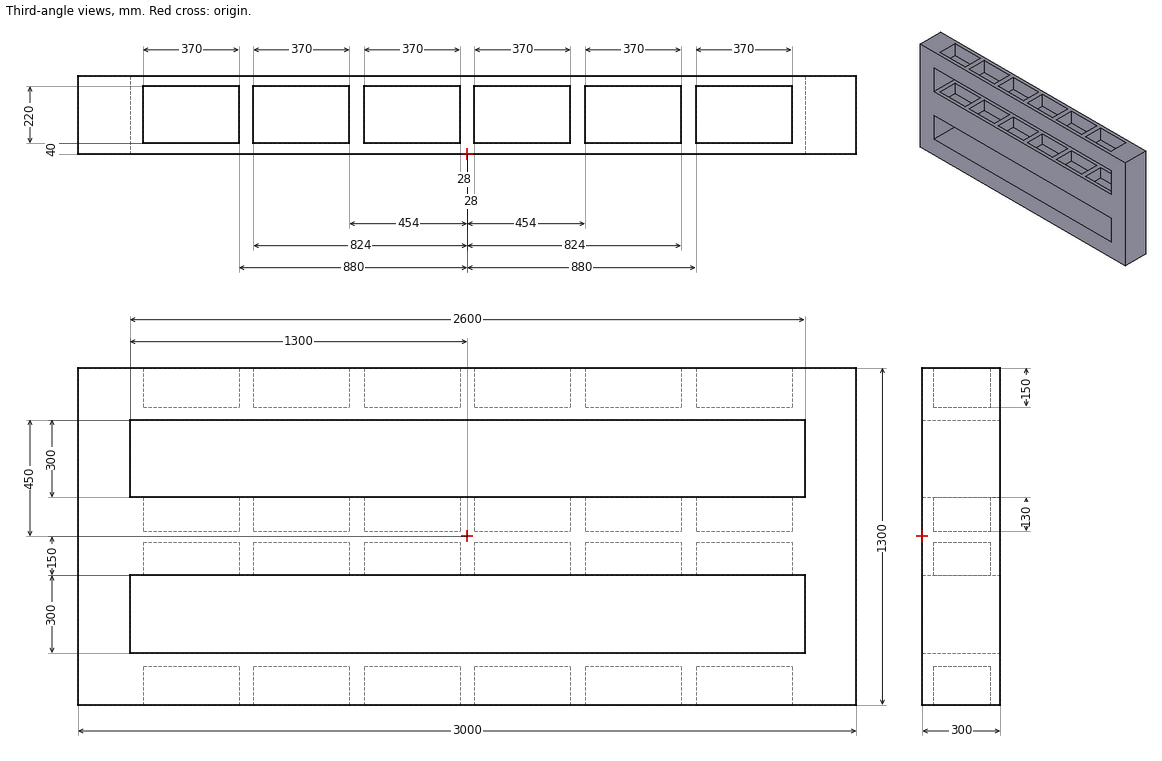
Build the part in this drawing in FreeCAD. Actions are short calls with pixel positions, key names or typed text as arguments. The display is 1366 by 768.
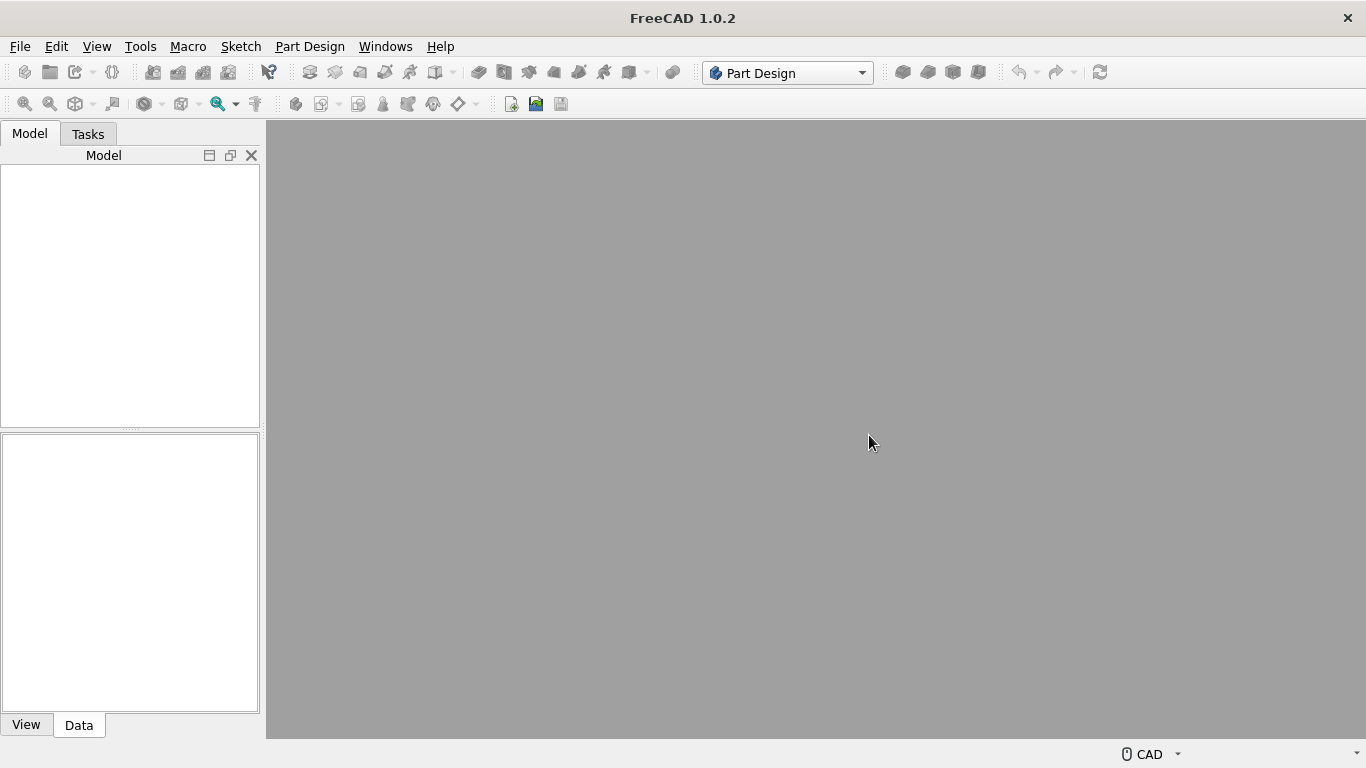
key(ctrl+n)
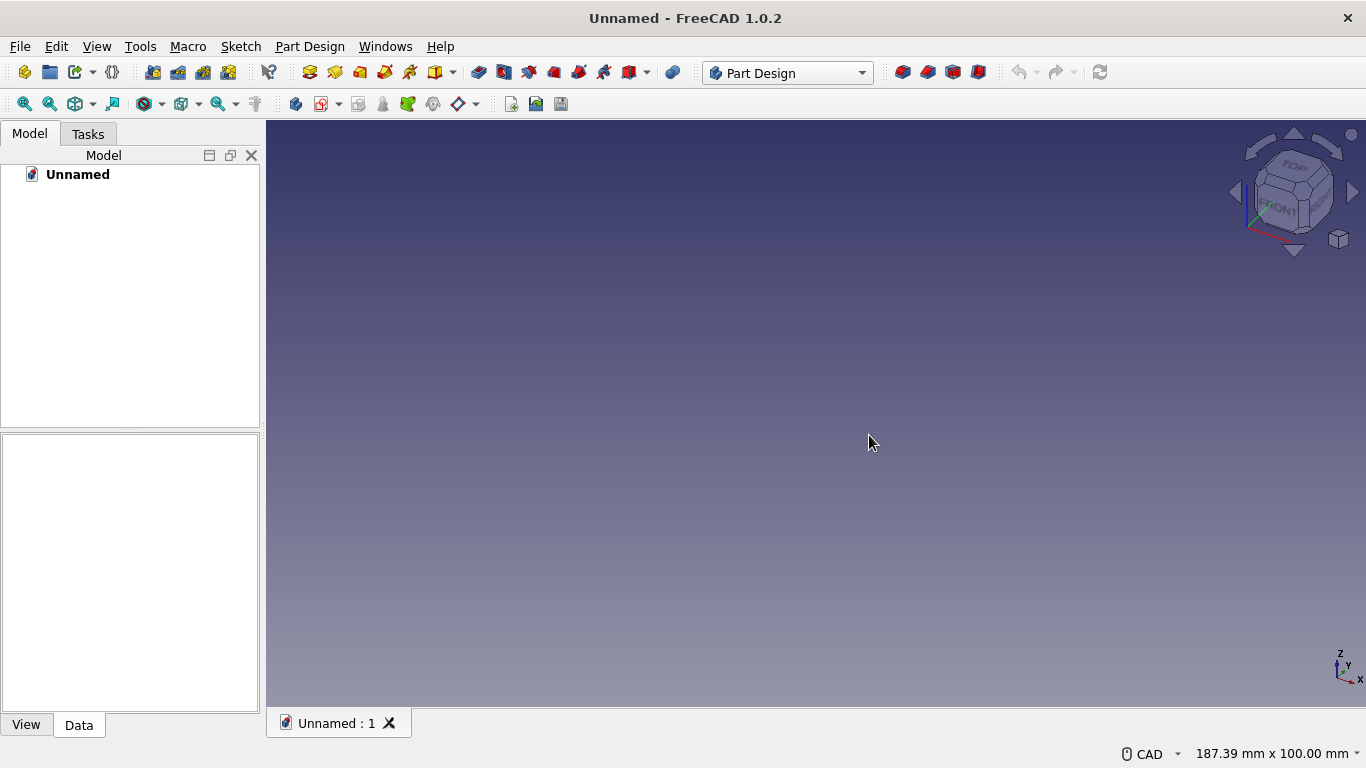
click(320, 104)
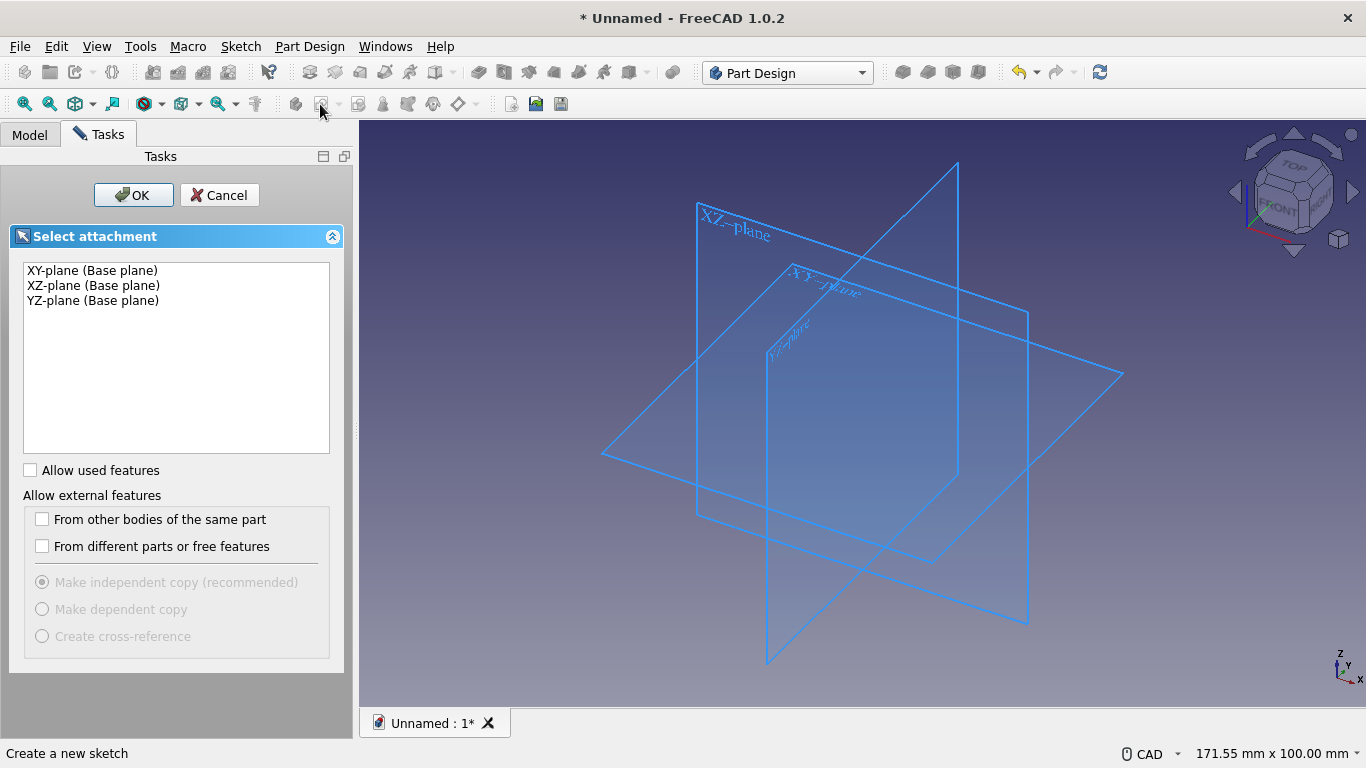
click(84, 286)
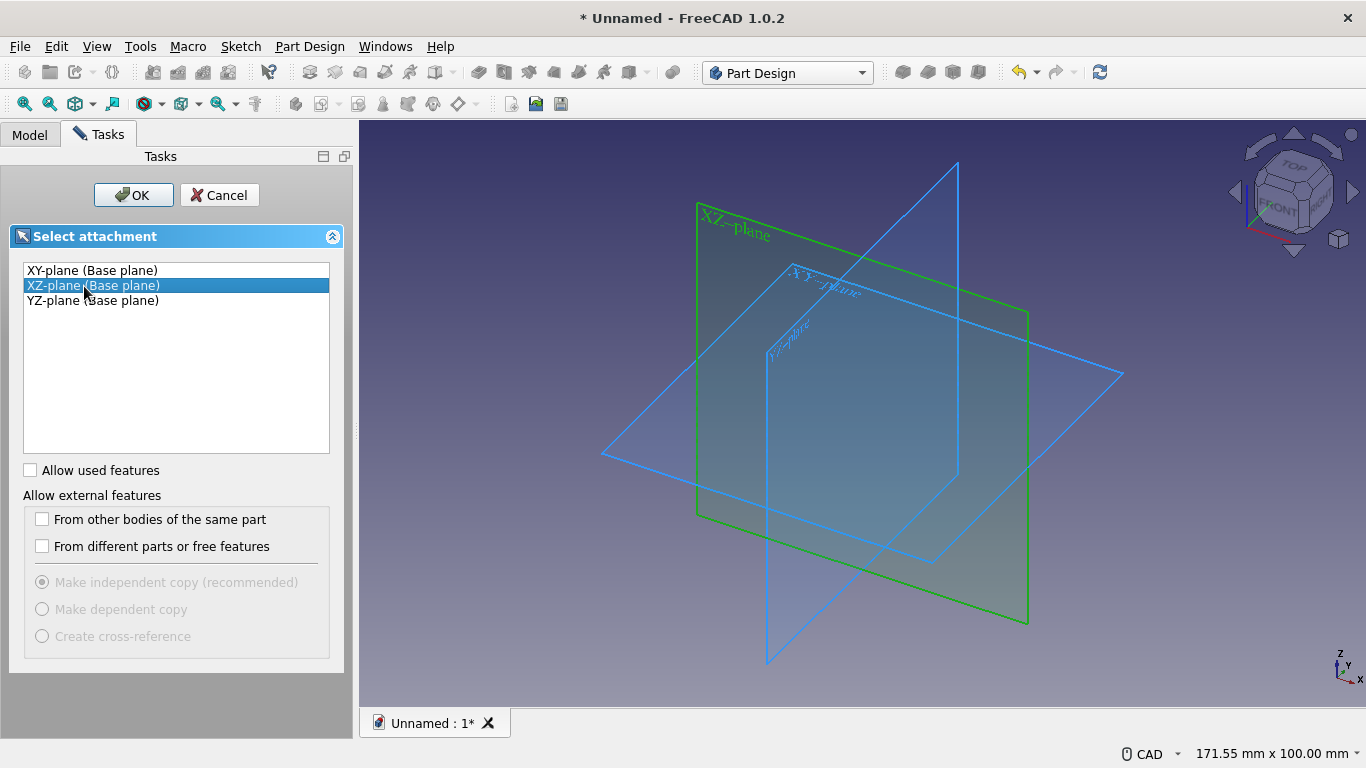
click(134, 195)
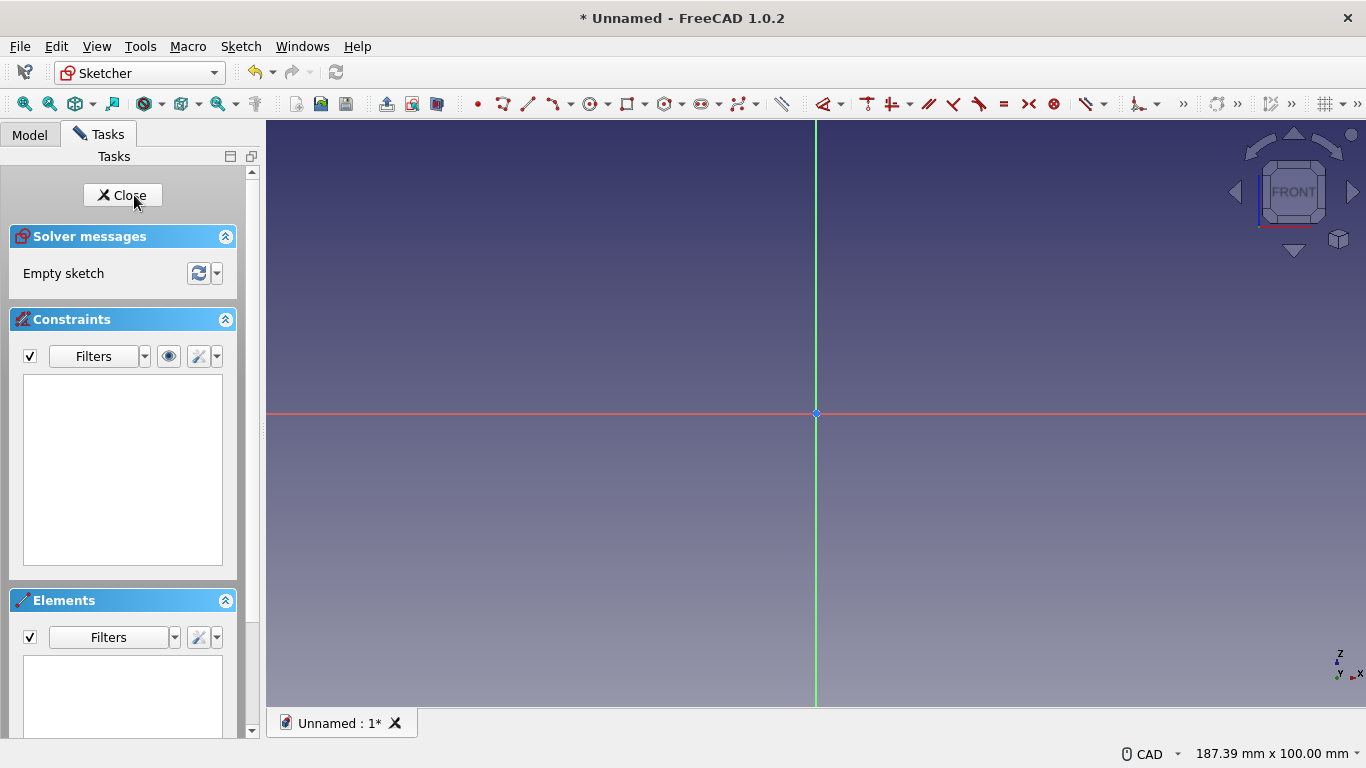
scroll(745, 414, down, 16)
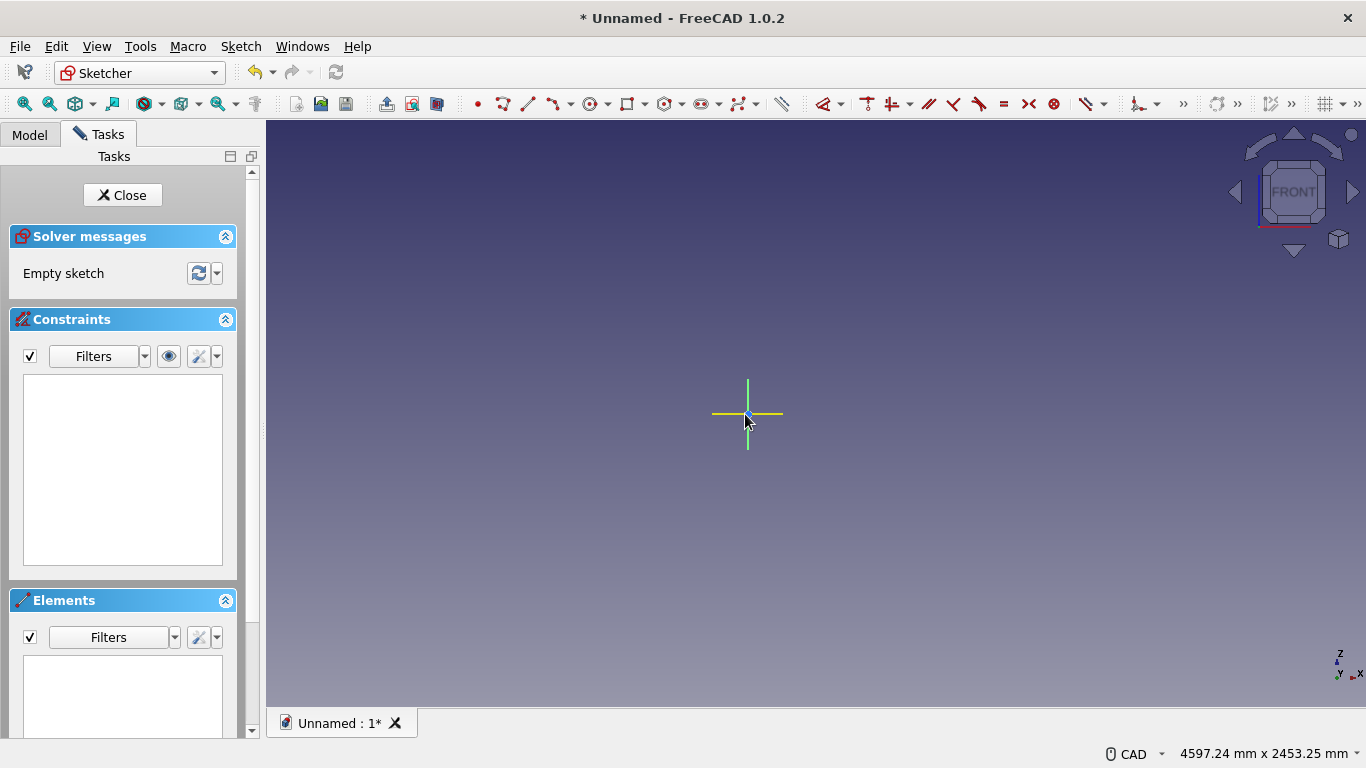
key(g)
key(v)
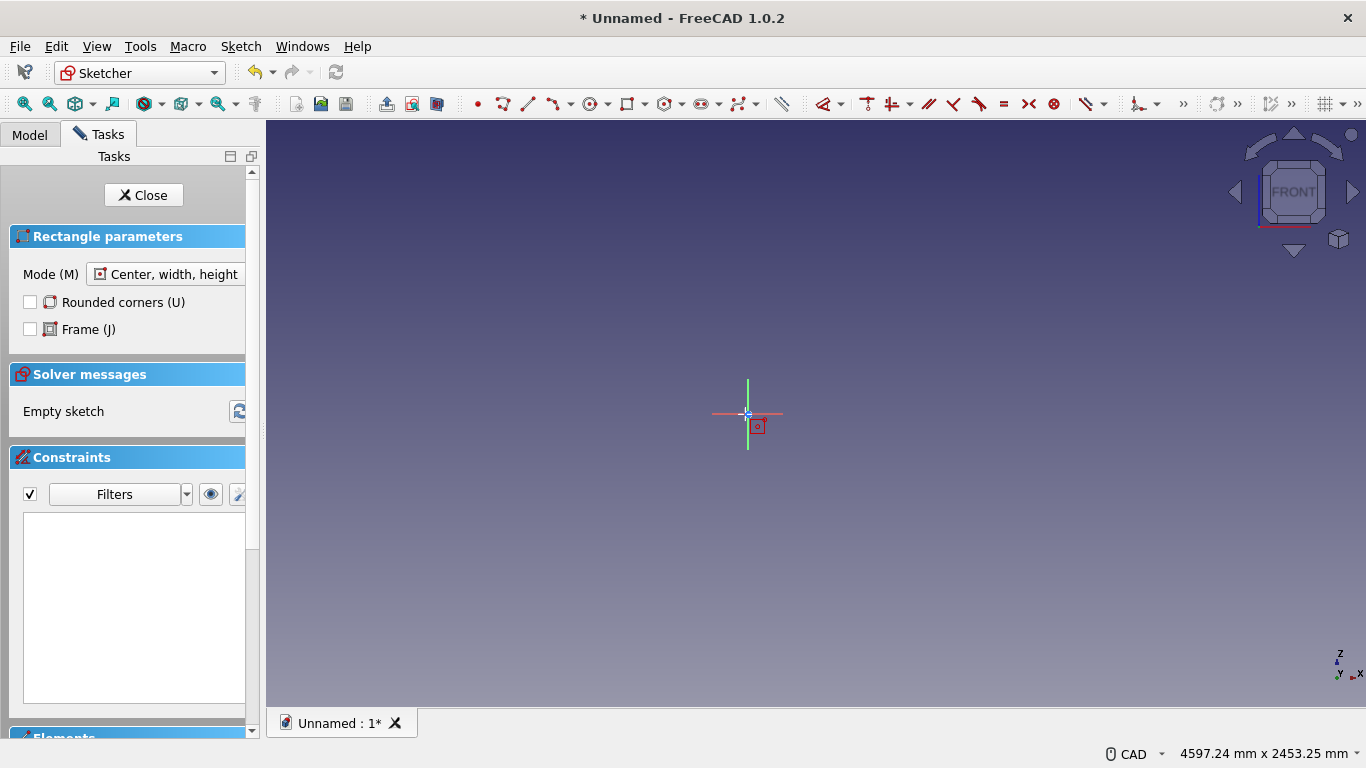
click(748, 414)
click(1107, 259)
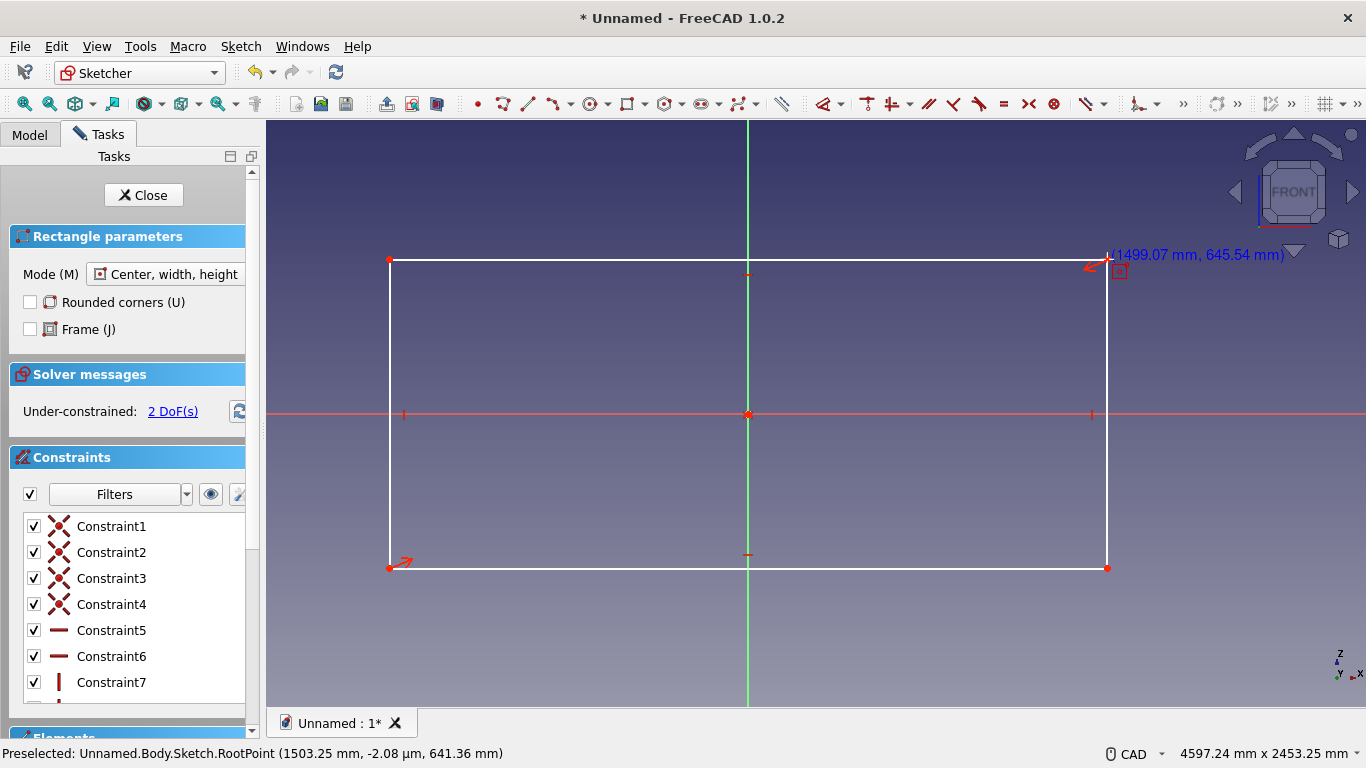
key(g)
key(r)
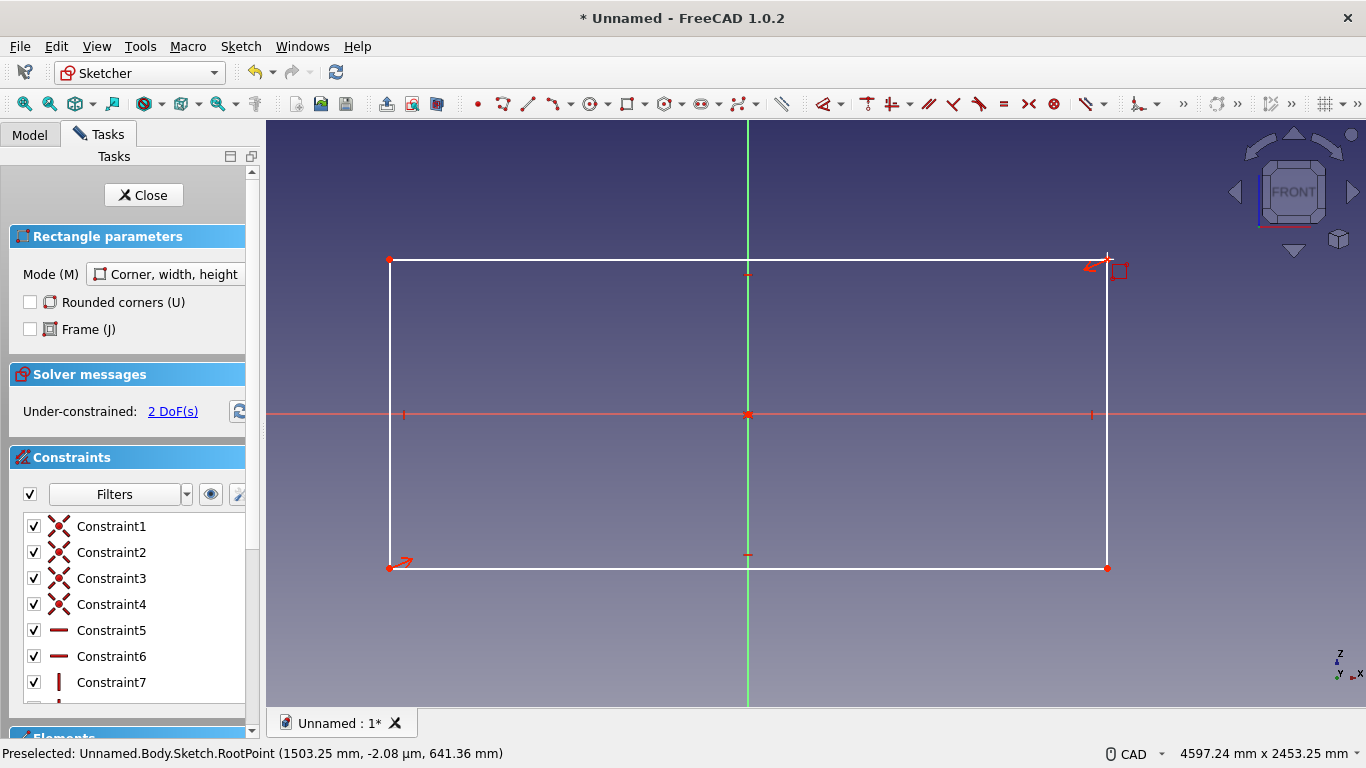
click(437, 307)
click(1059, 379)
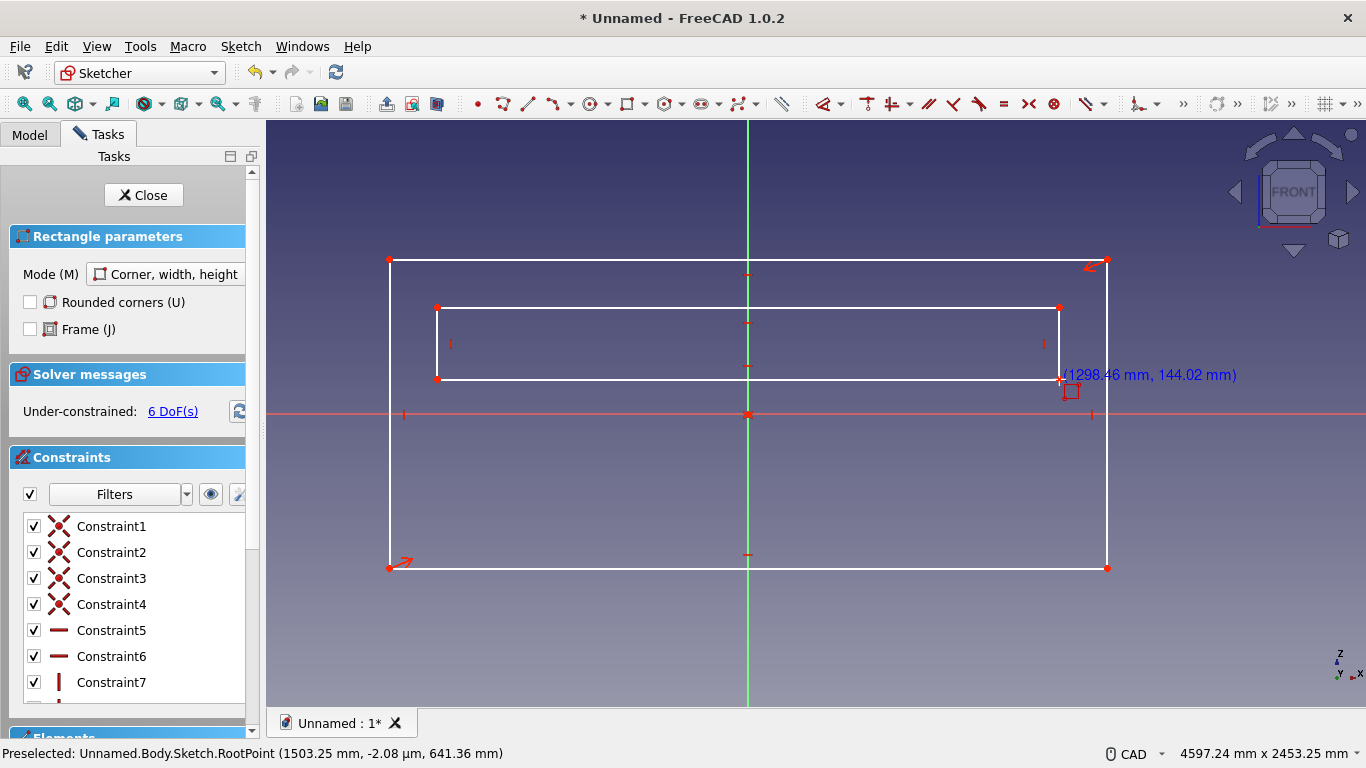
click(437, 450)
click(1059, 522)
key(Escape)